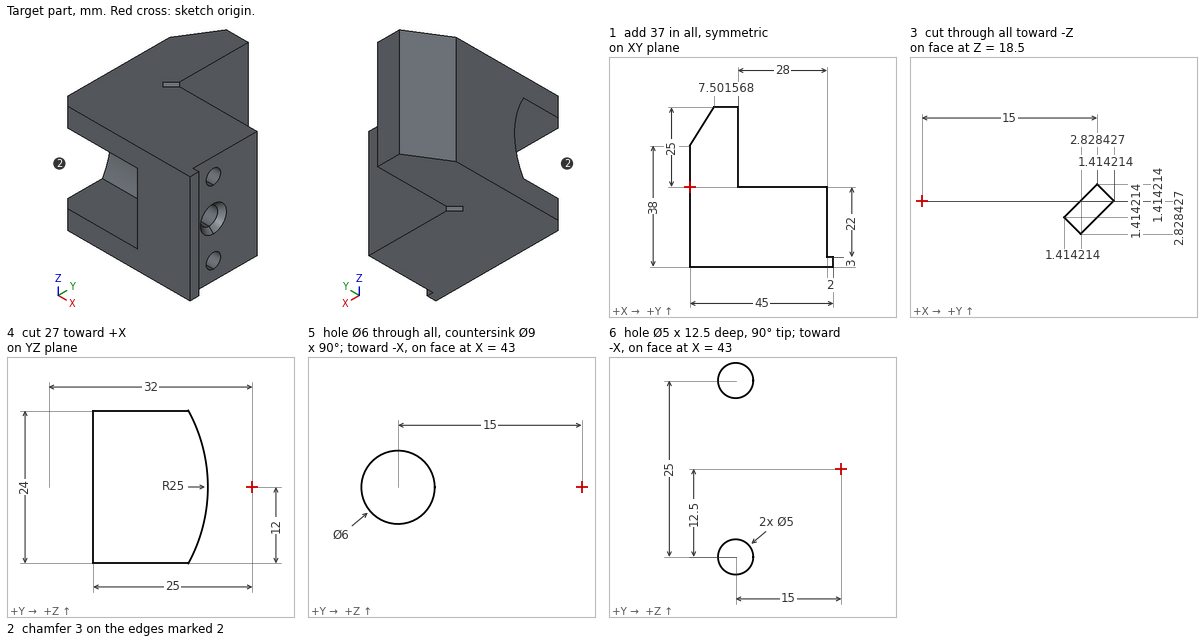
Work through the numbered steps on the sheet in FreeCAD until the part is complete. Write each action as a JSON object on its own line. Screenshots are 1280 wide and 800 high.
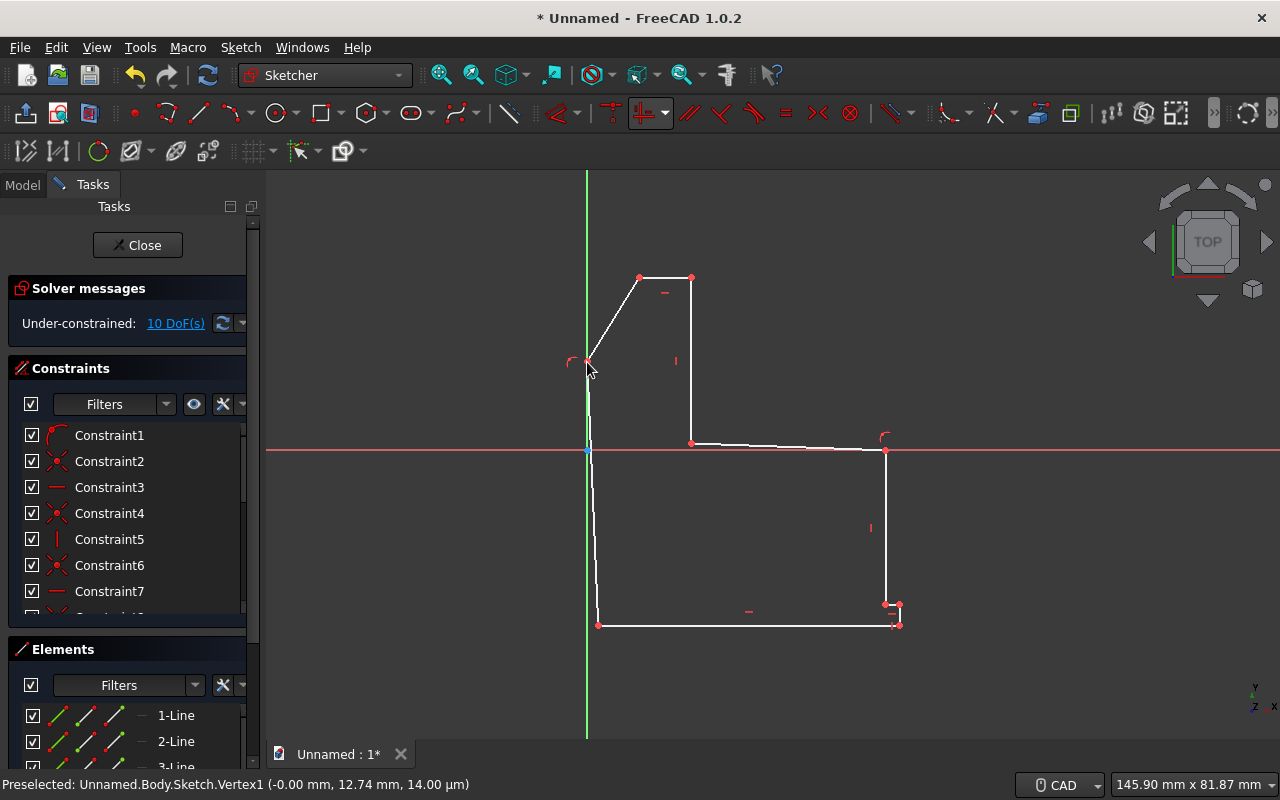
{"action": "scroll", "coordinate": [591, 441], "scroll_direction": "up", "scroll_amount": 2}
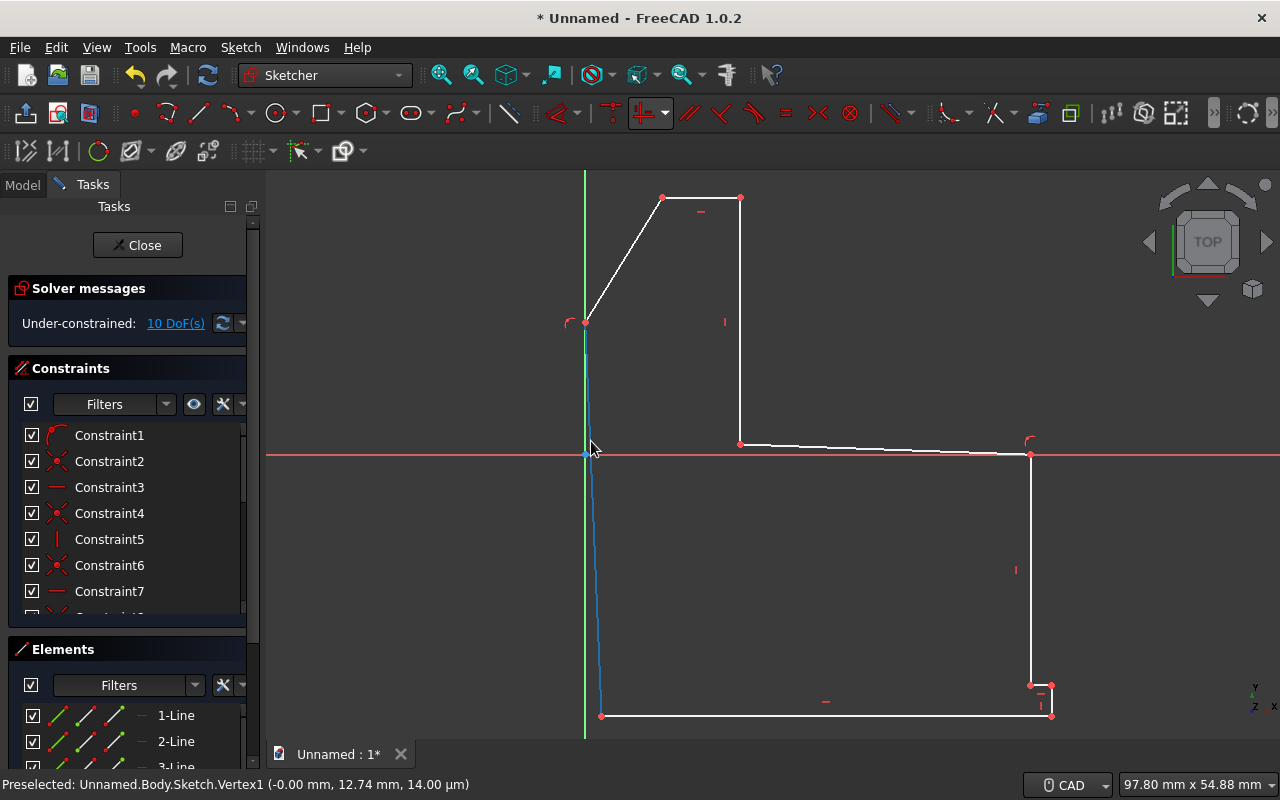
{"action": "left_click", "coordinate": [590, 441]}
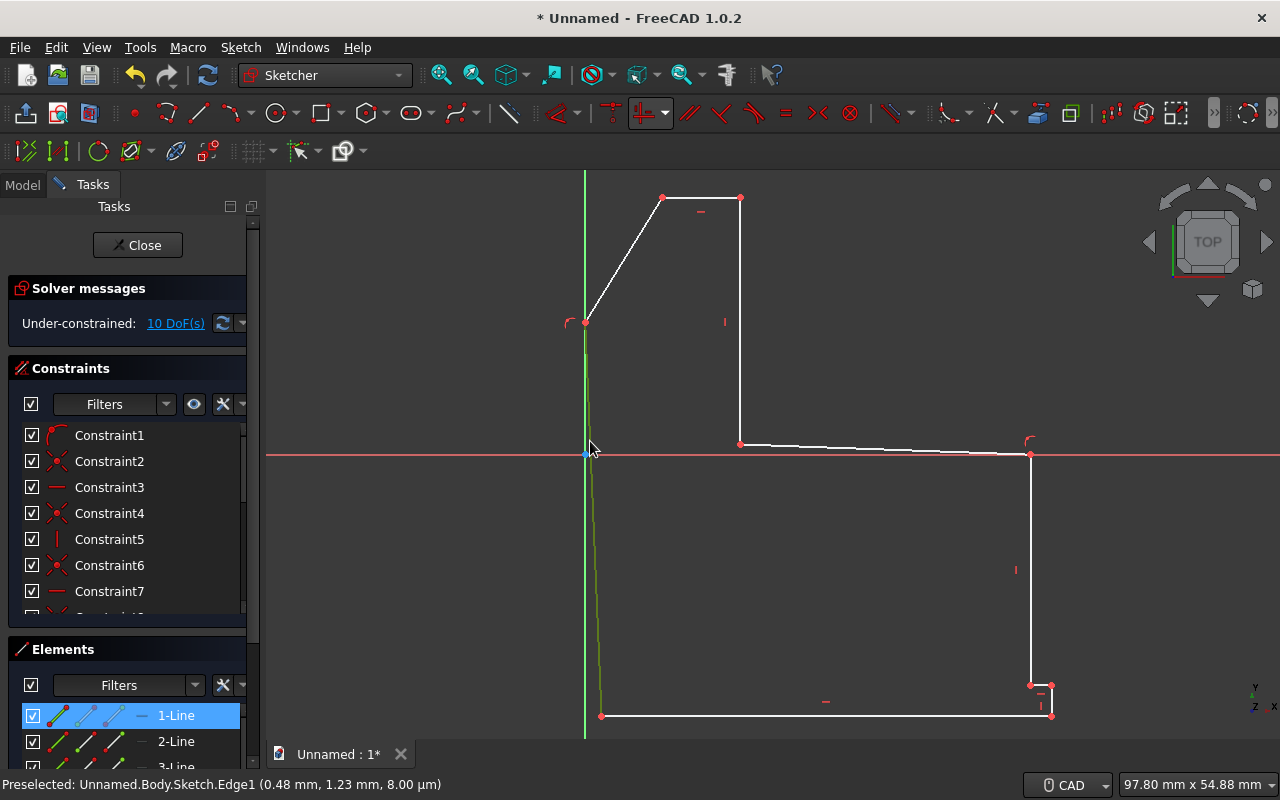
{"action": "left_click", "coordinate": [668, 114]}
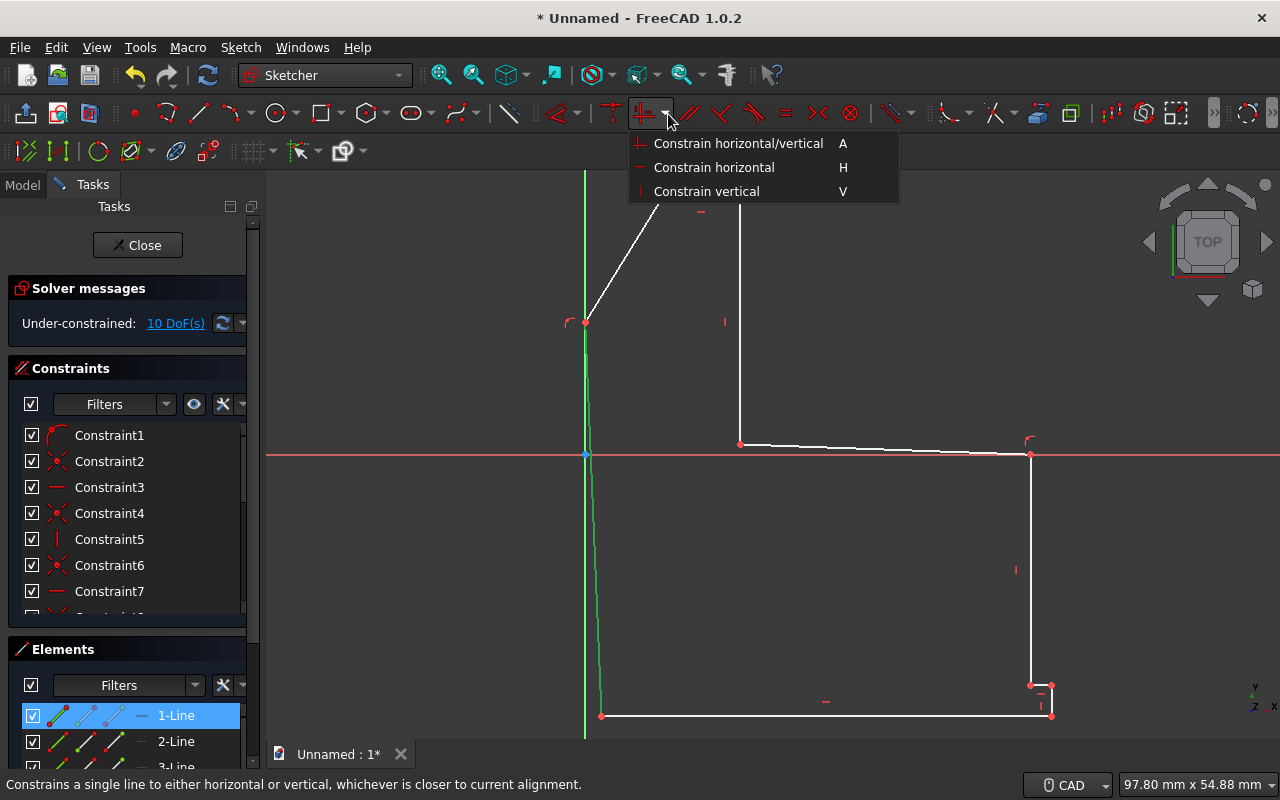
{"action": "left_click", "coordinate": [764, 191]}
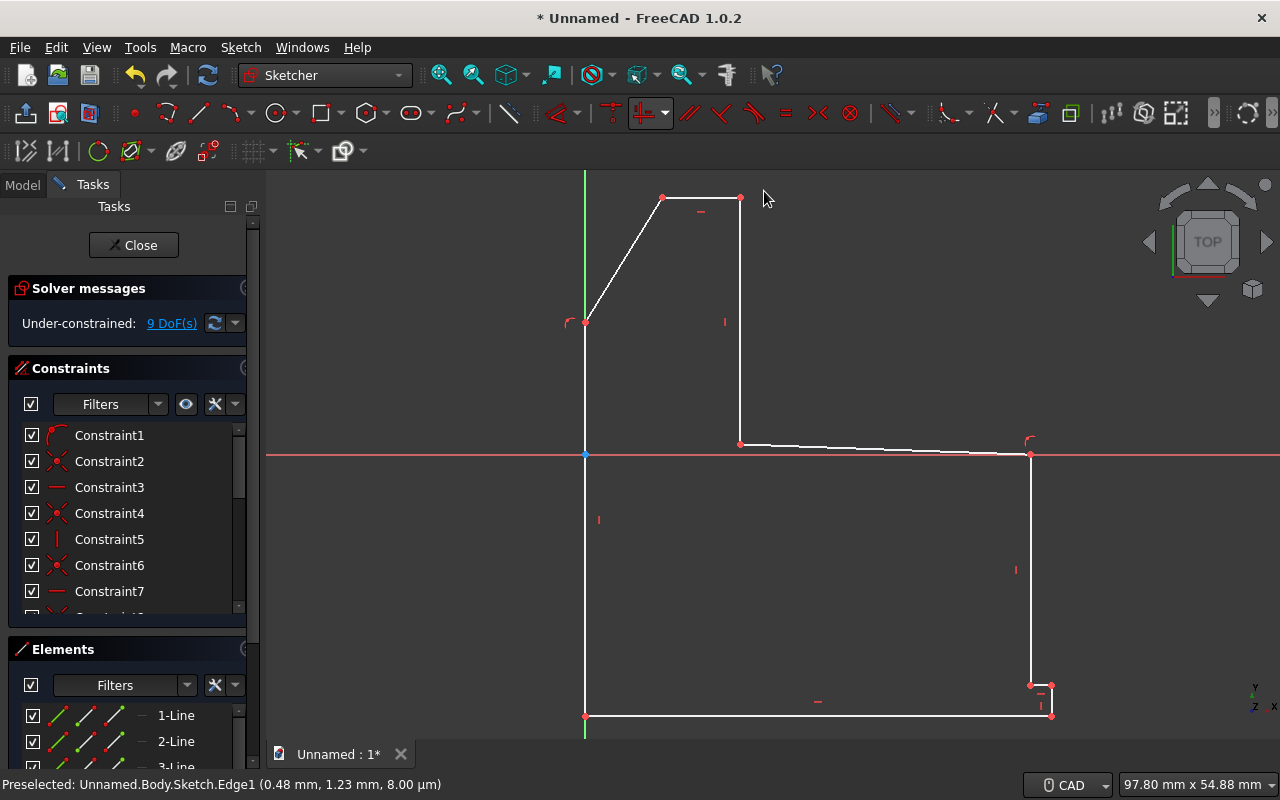
{"action": "left_click", "coordinate": [944, 452]}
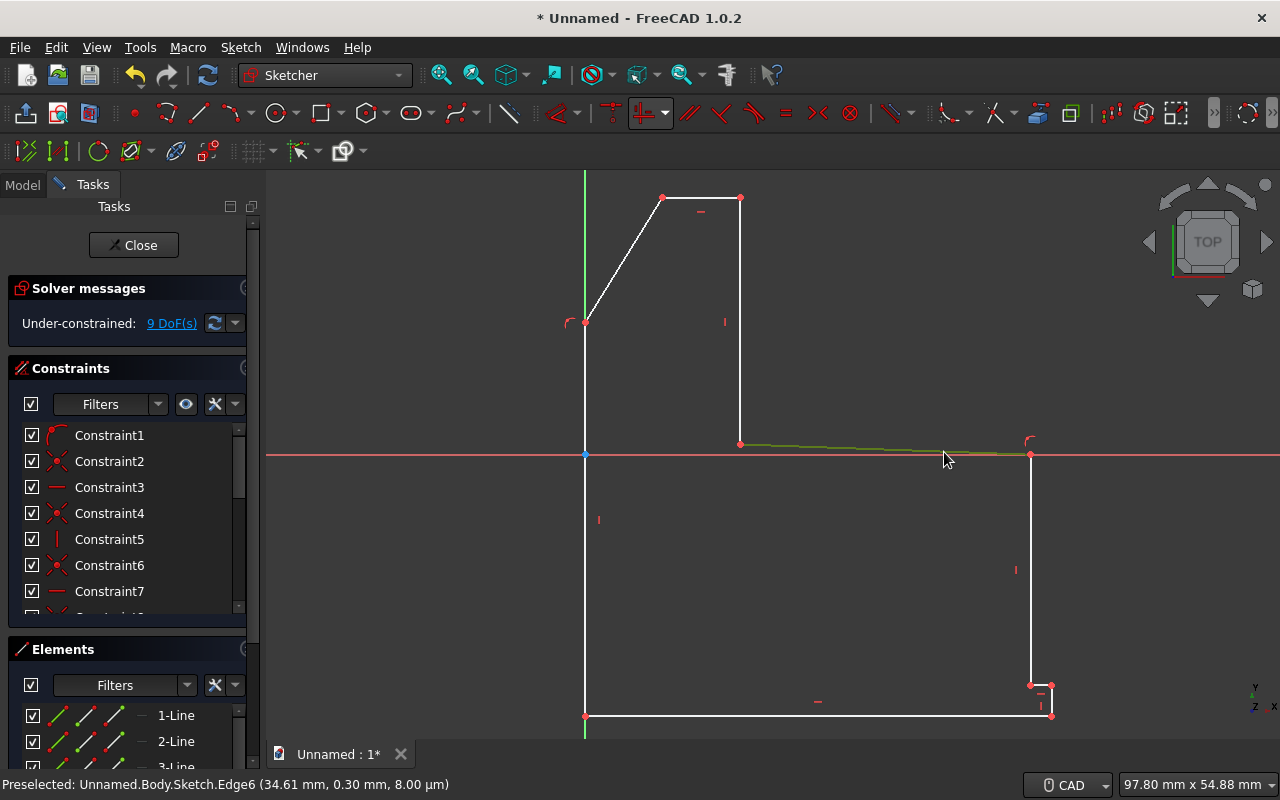
{"action": "key", "text": "h"}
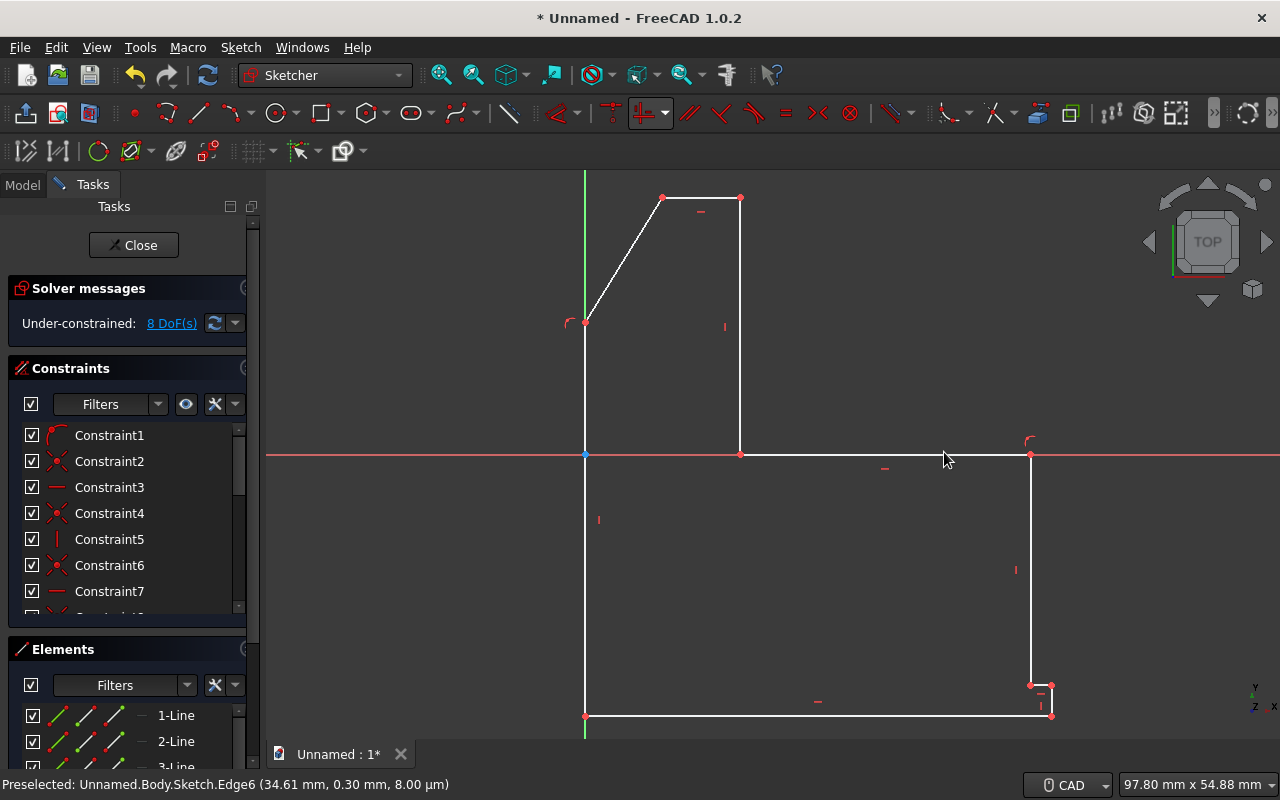
{"action": "left_click", "coordinate": [556, 114]}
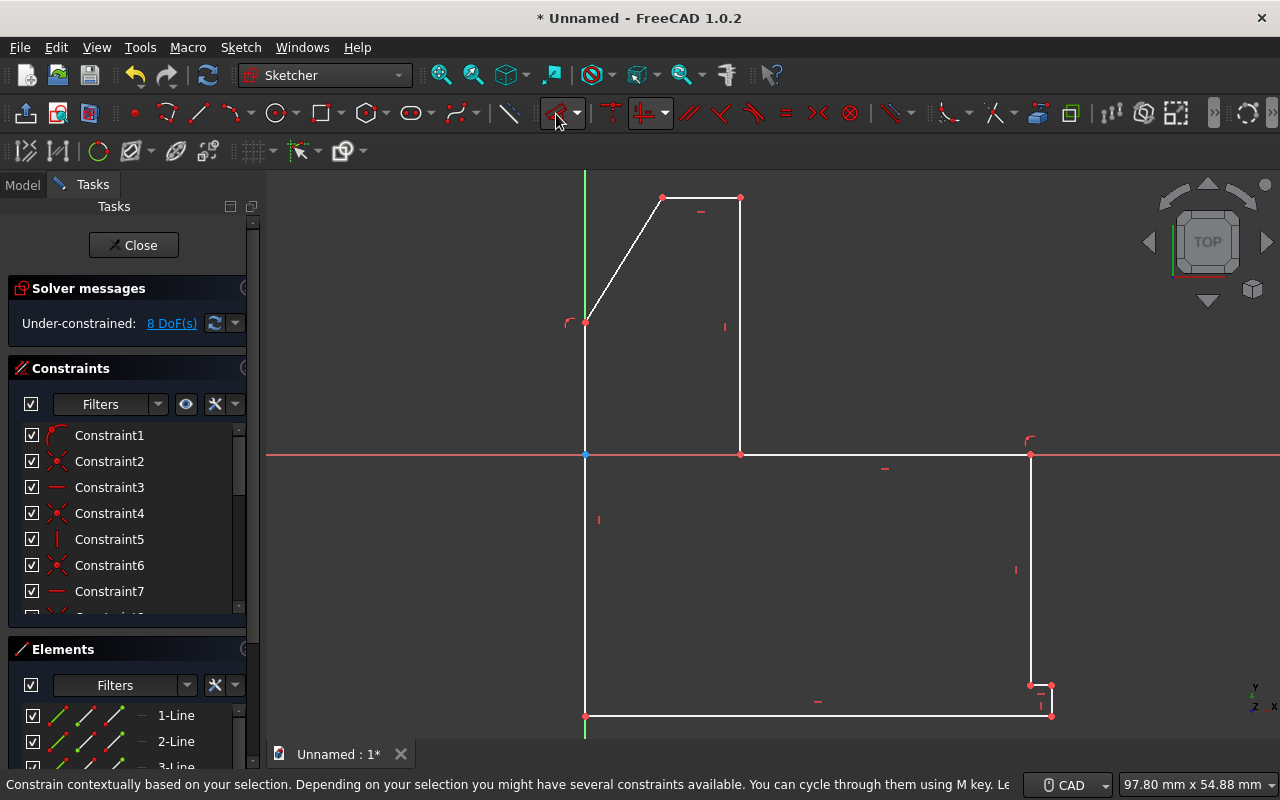
{"action": "scroll", "coordinate": [1052, 707], "scroll_direction": "up", "scroll_amount": 2}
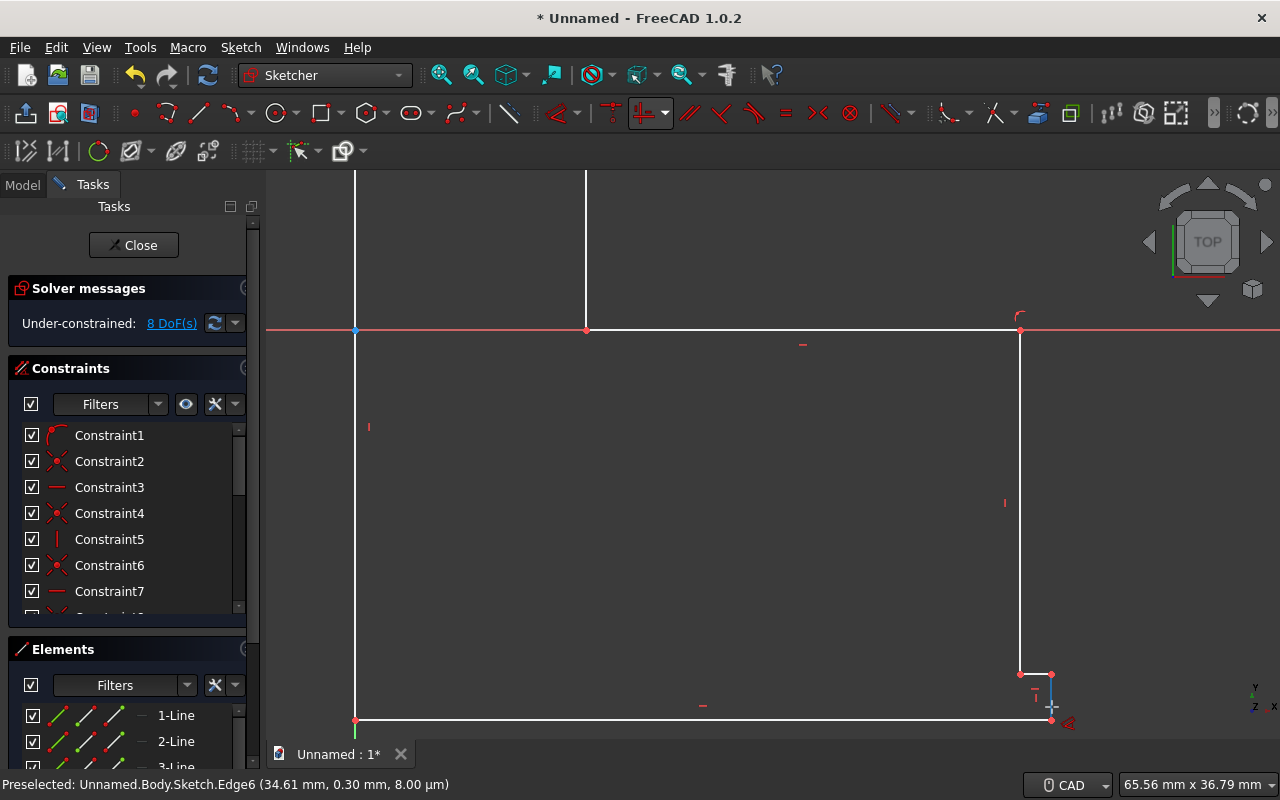
{"action": "left_click", "coordinate": [1051, 706]}
{"action": "left_click", "coordinate": [1085, 693]}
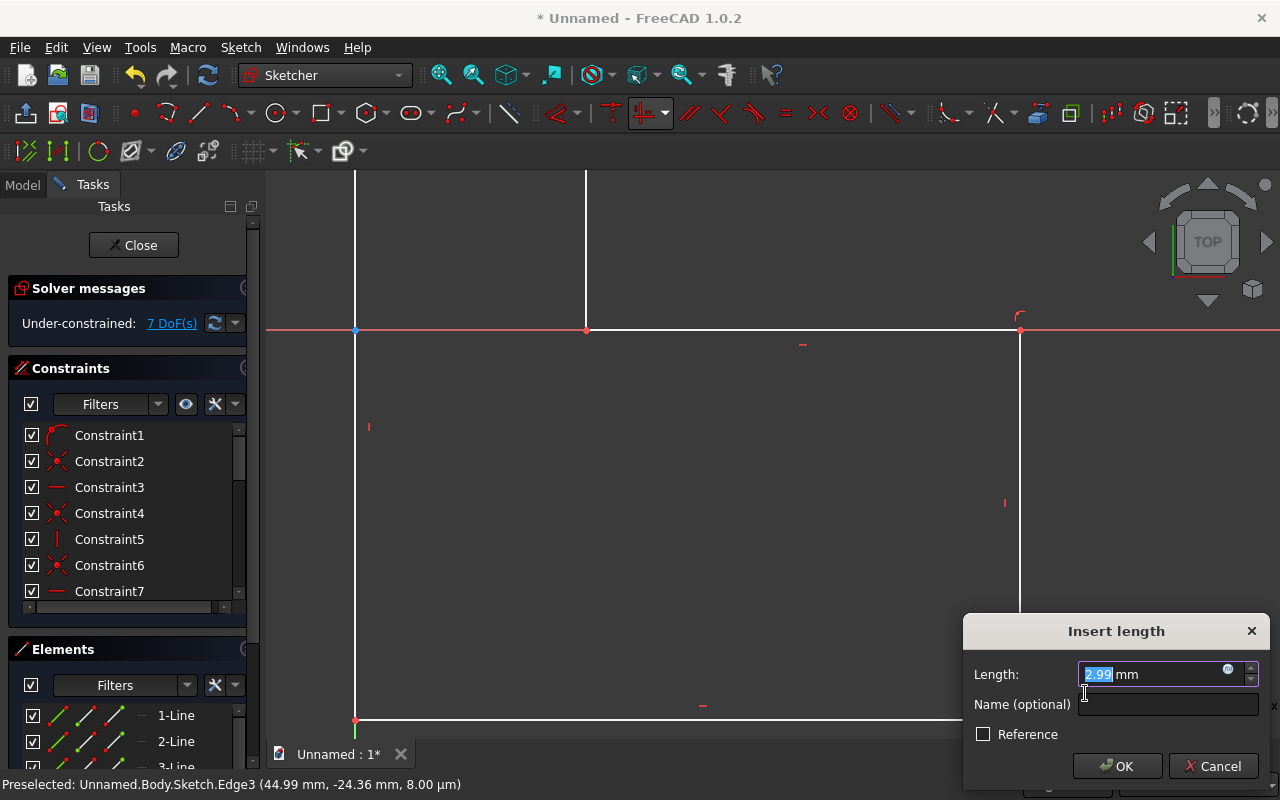
{"action": "type", "text": "3"}
{"action": "key", "text": "Return"}